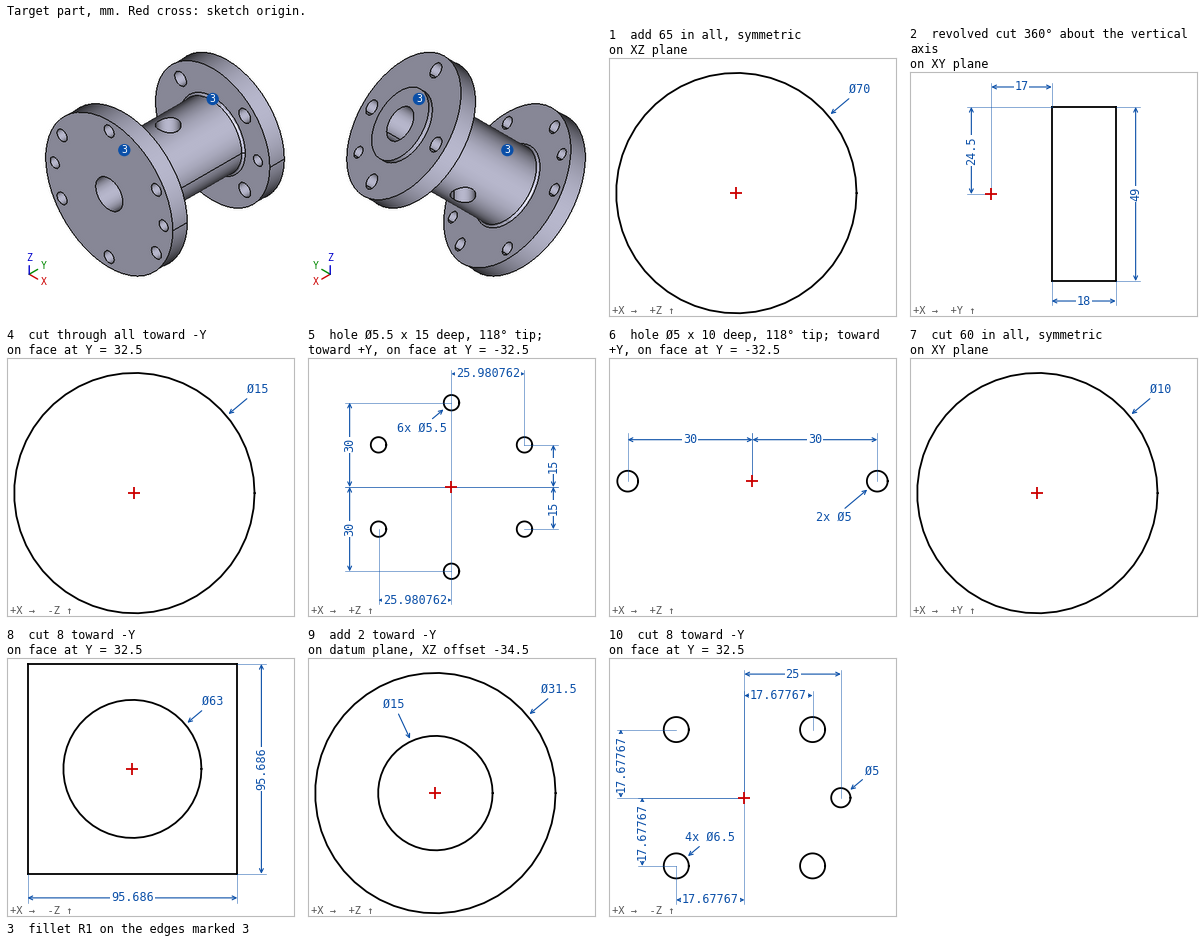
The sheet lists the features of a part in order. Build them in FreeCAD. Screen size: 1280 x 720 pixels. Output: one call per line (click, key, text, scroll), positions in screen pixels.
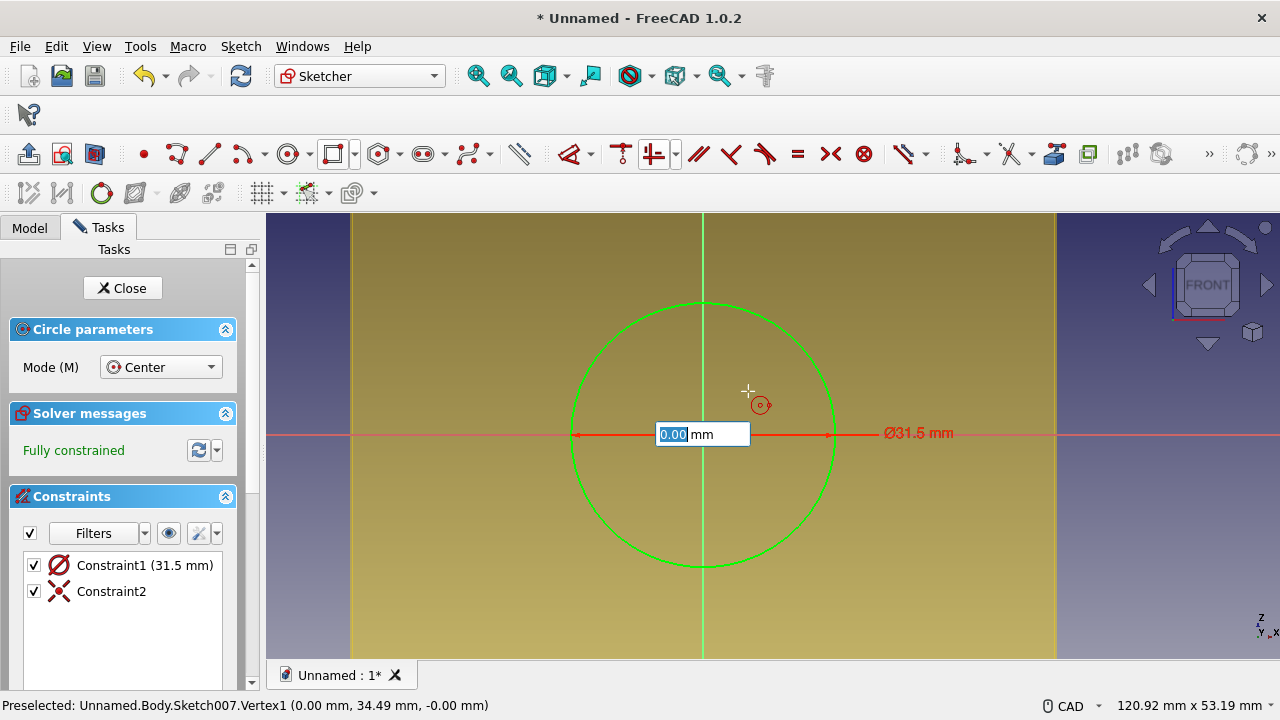
text(15)
key(Return)
key(Escape)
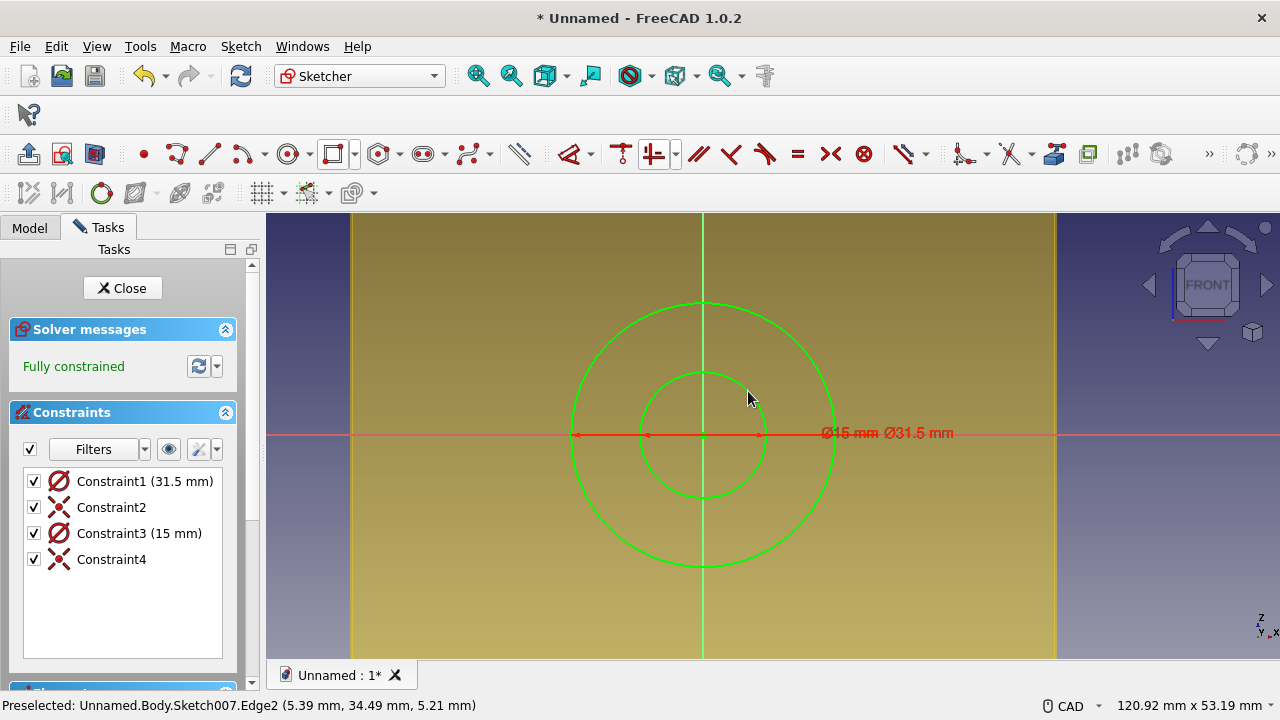
click(123, 288)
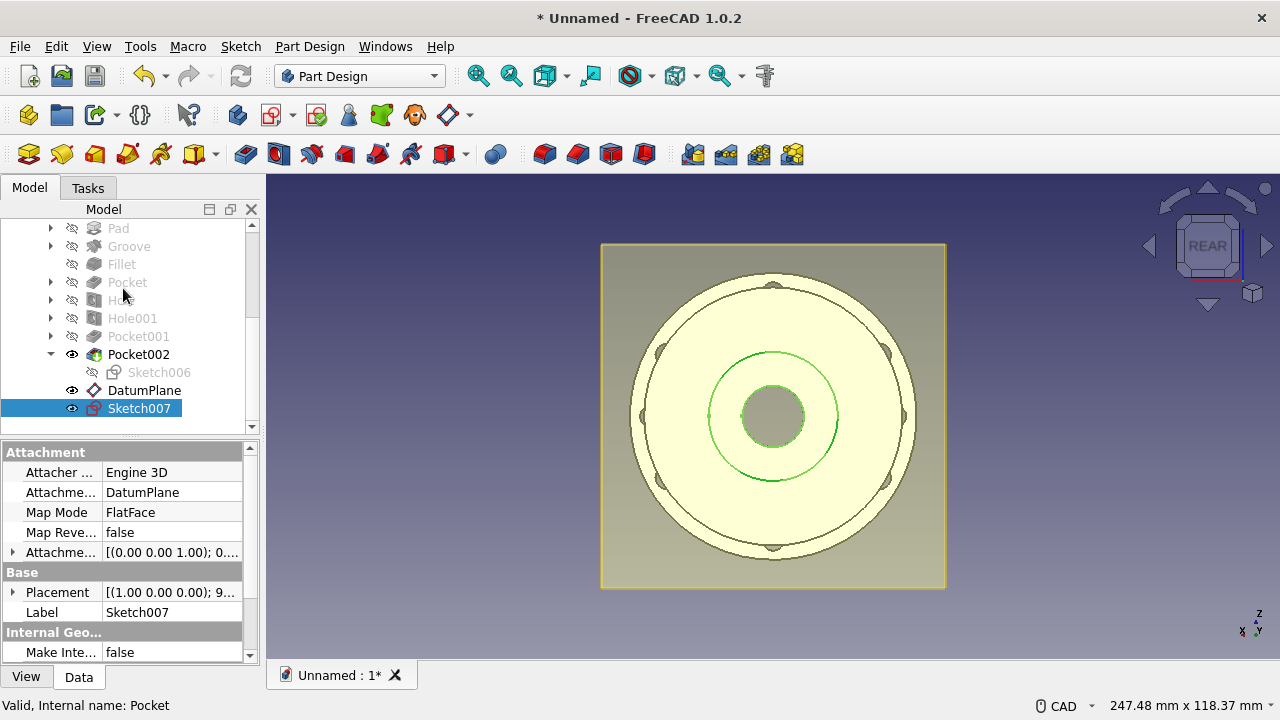
click(29, 154)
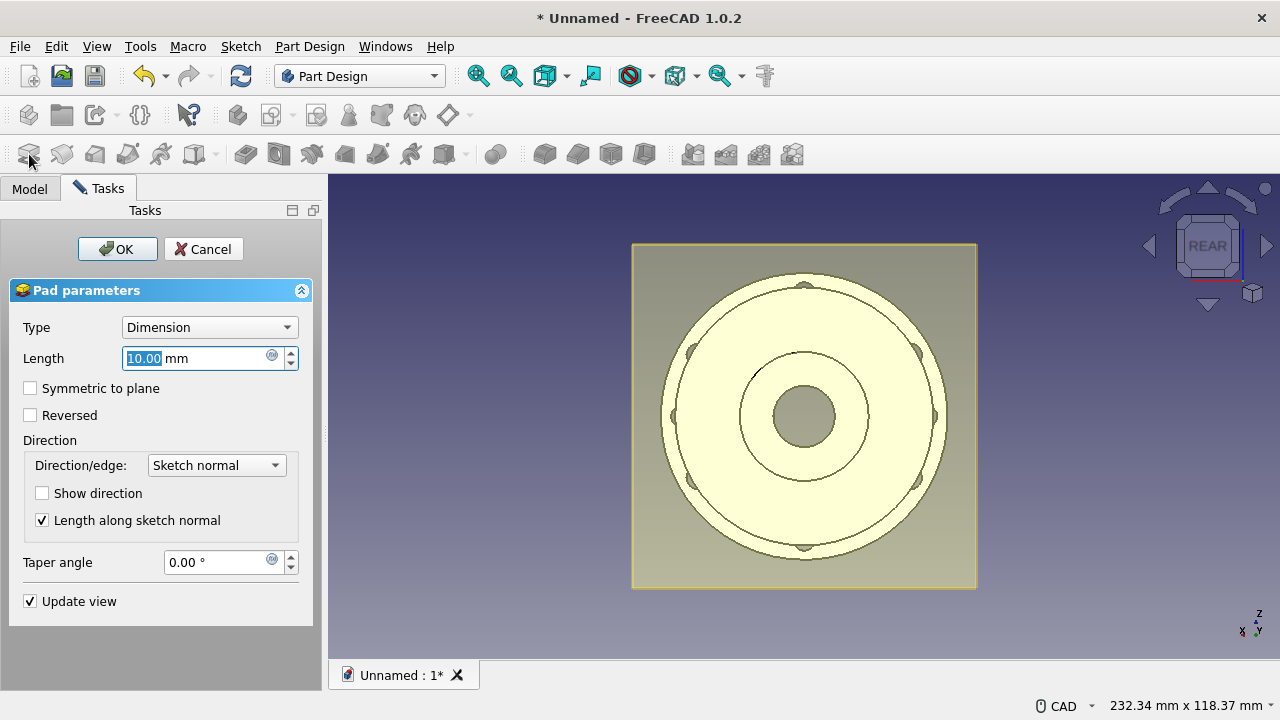
text(2)
key(Tab)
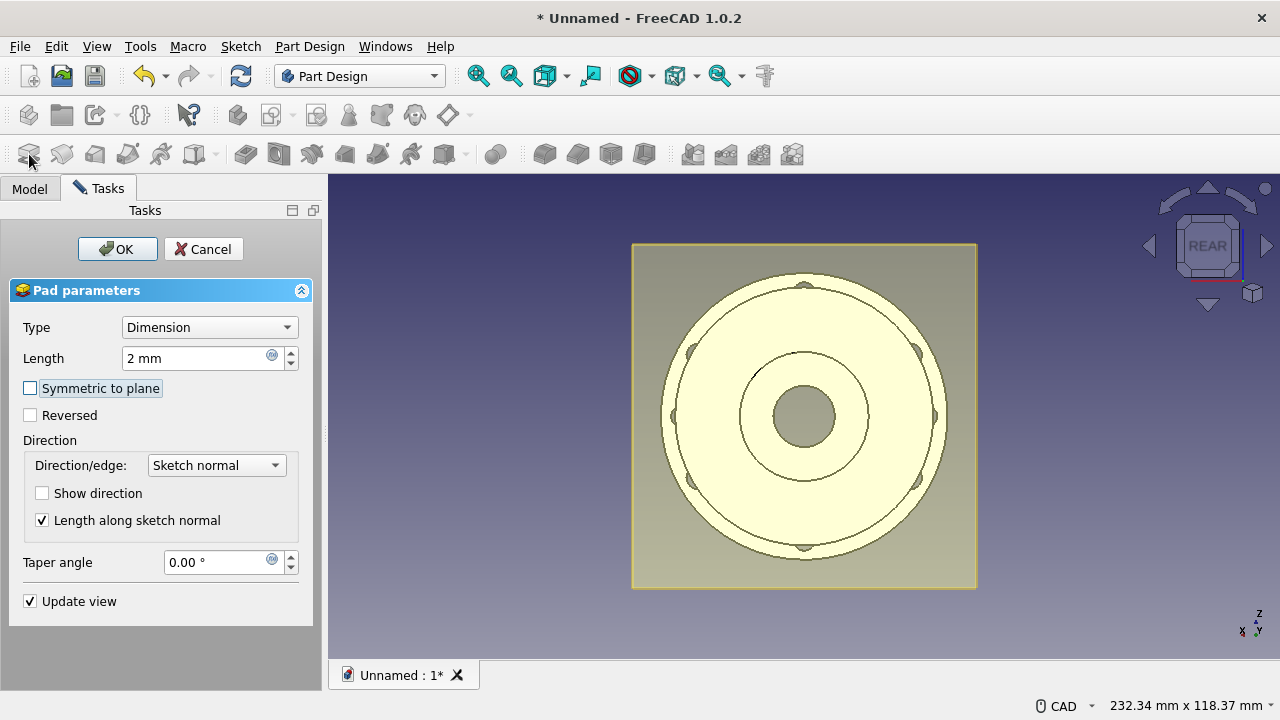
click(118, 249)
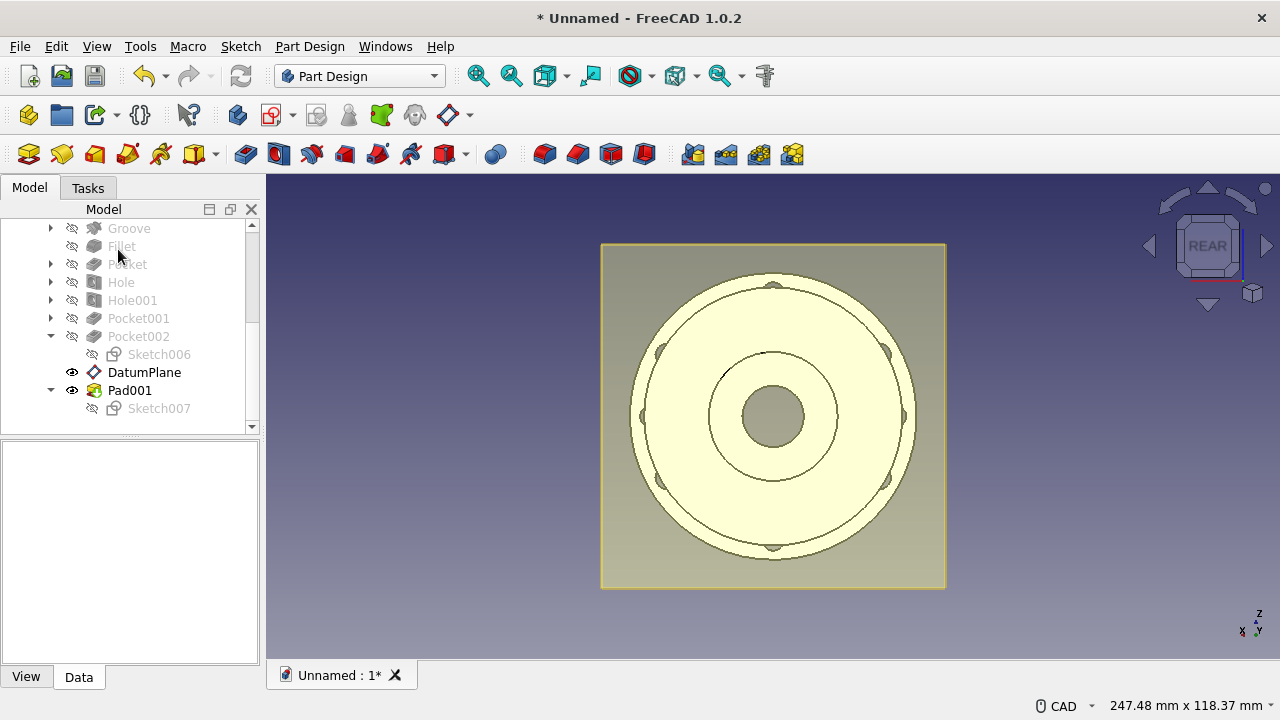
click(117, 372)
key(space)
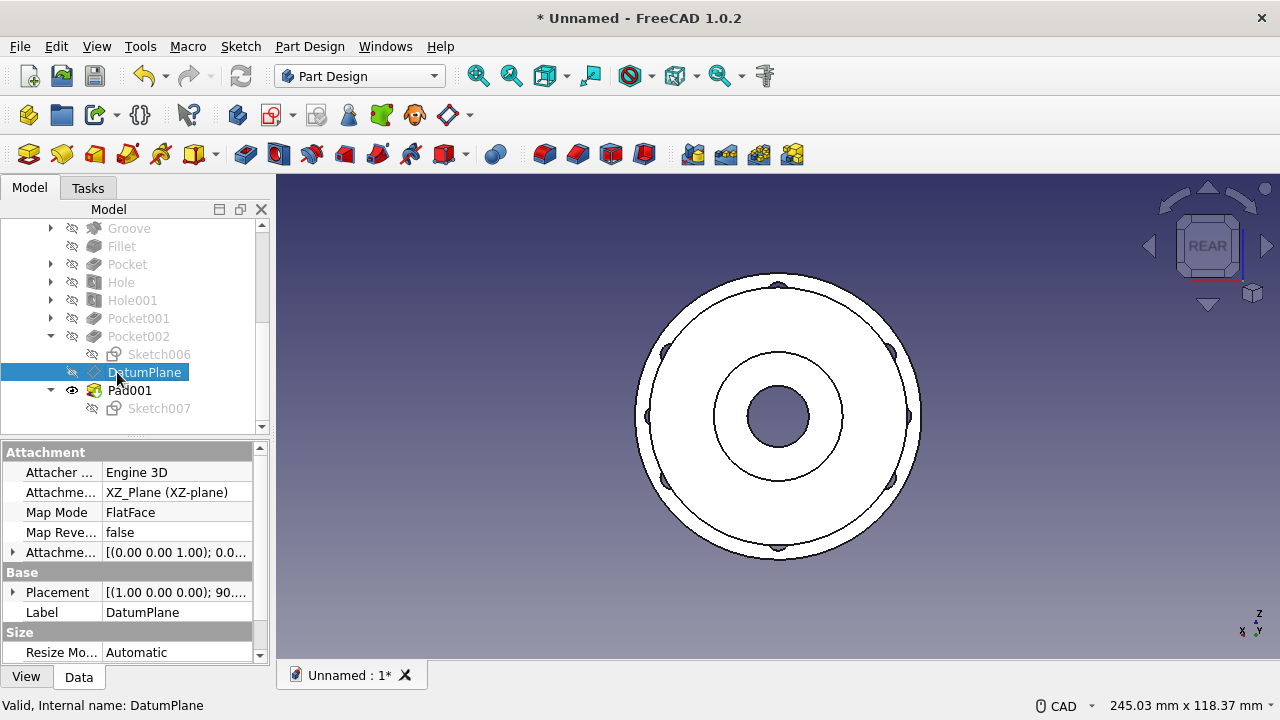
click(852, 342)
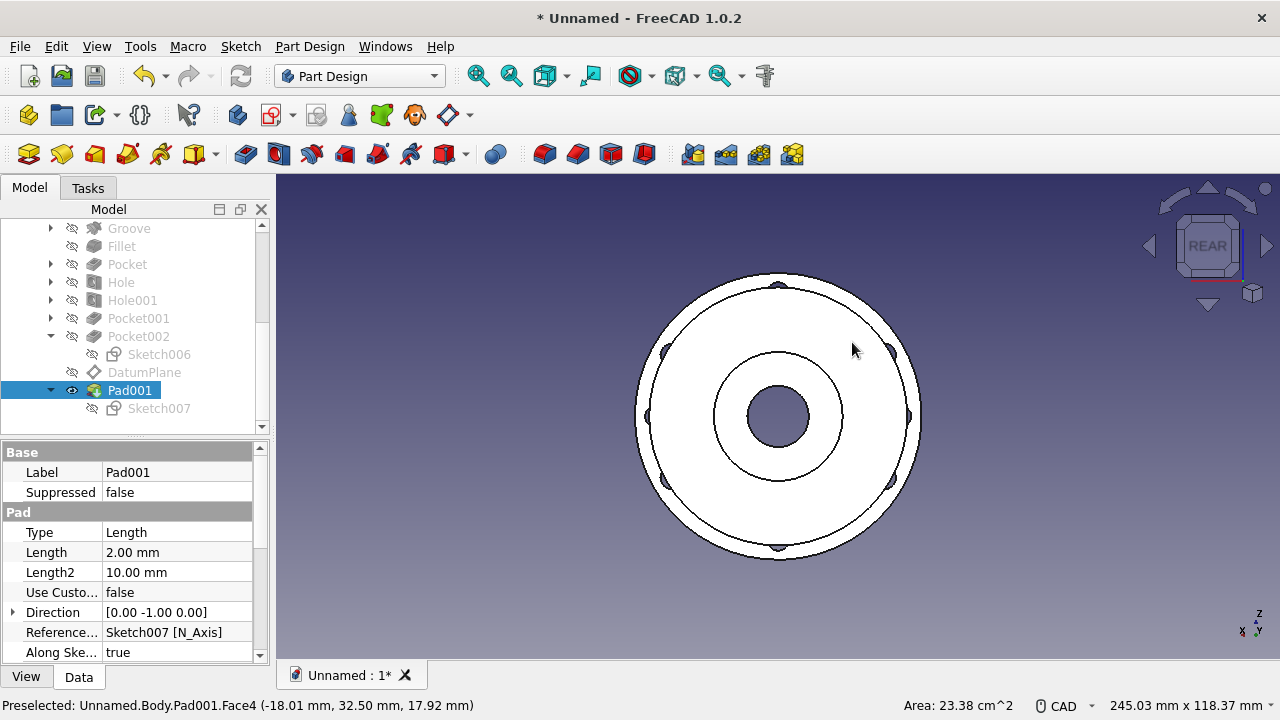
click(270, 116)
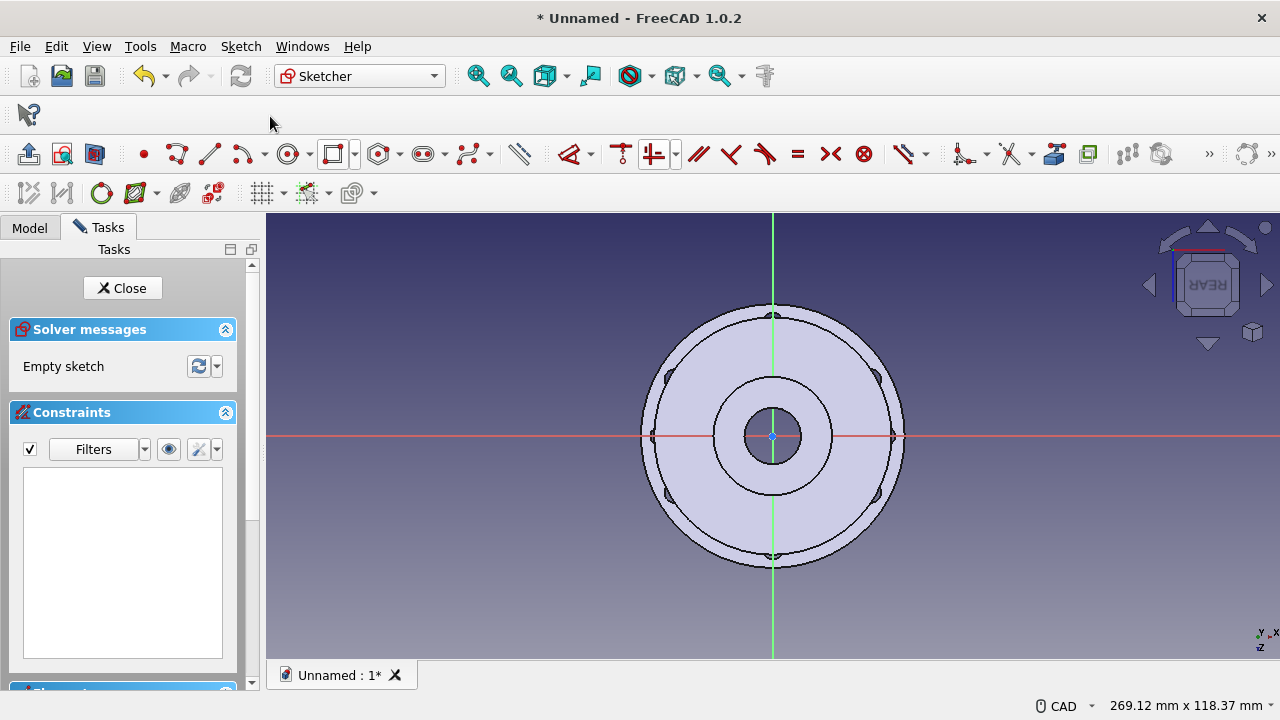
click(95, 154)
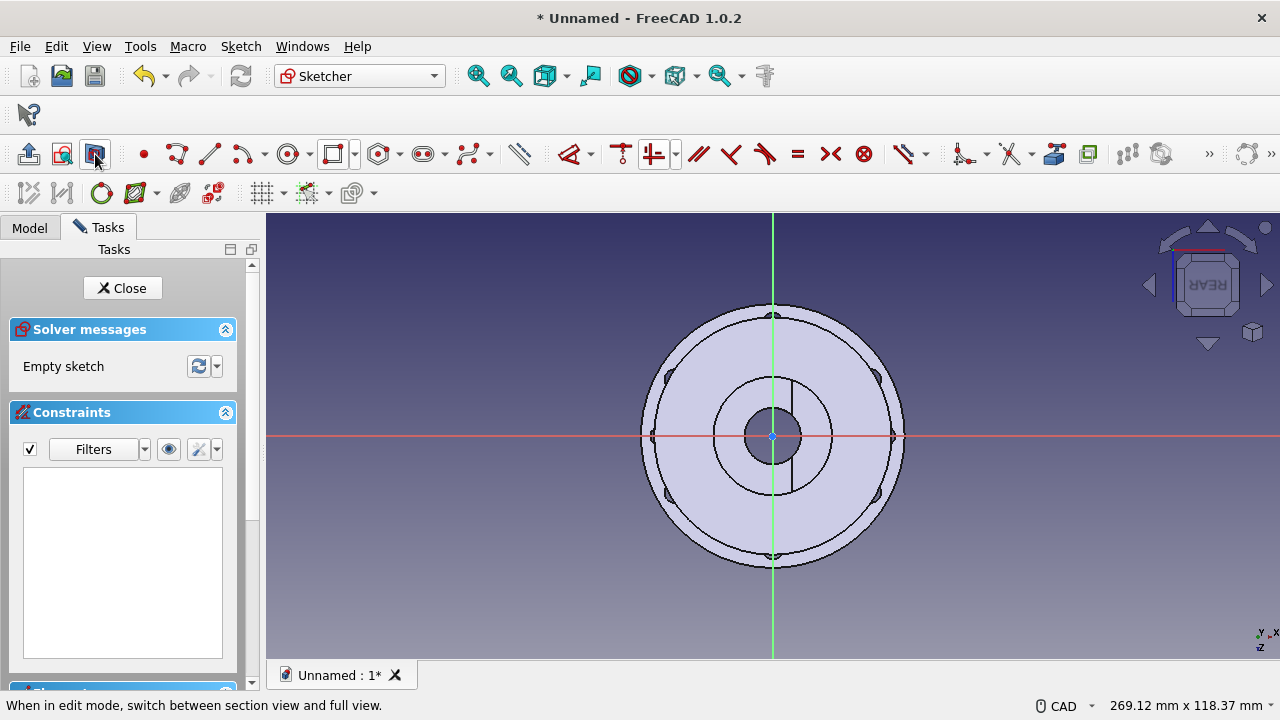
scroll(883, 436, up, 3)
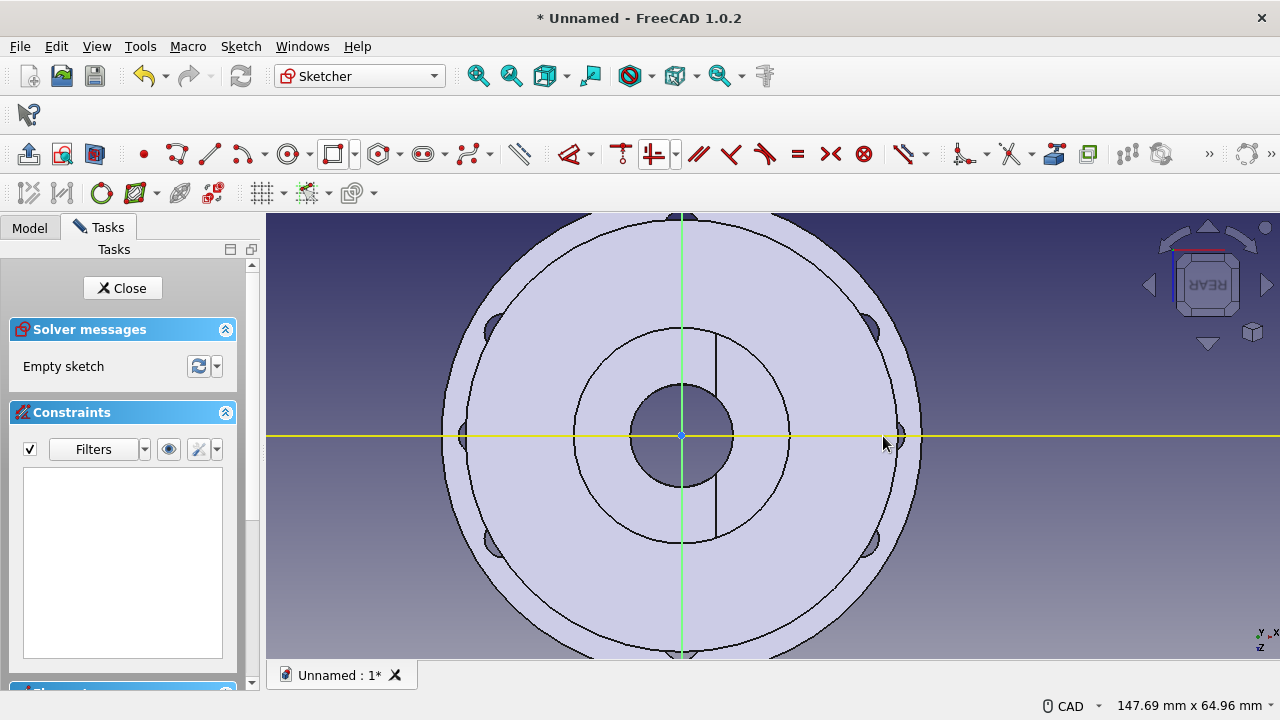
click(288, 154)